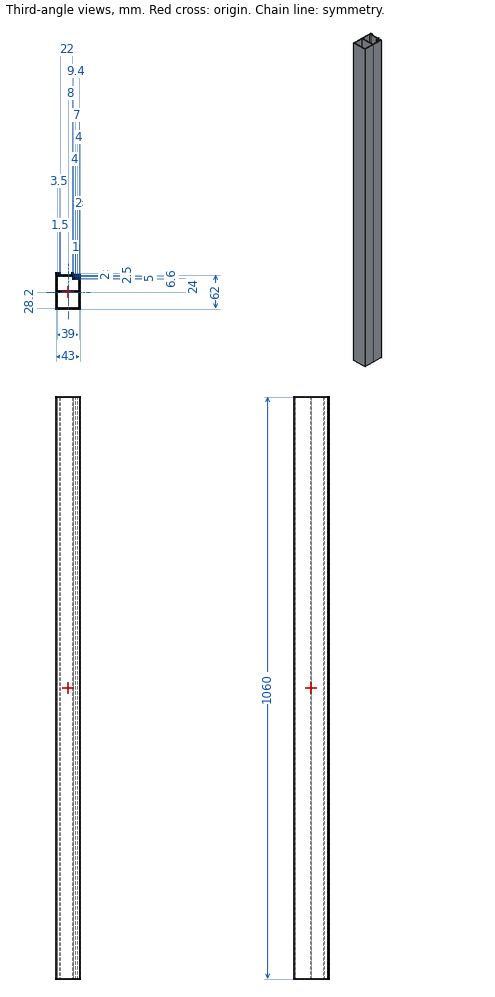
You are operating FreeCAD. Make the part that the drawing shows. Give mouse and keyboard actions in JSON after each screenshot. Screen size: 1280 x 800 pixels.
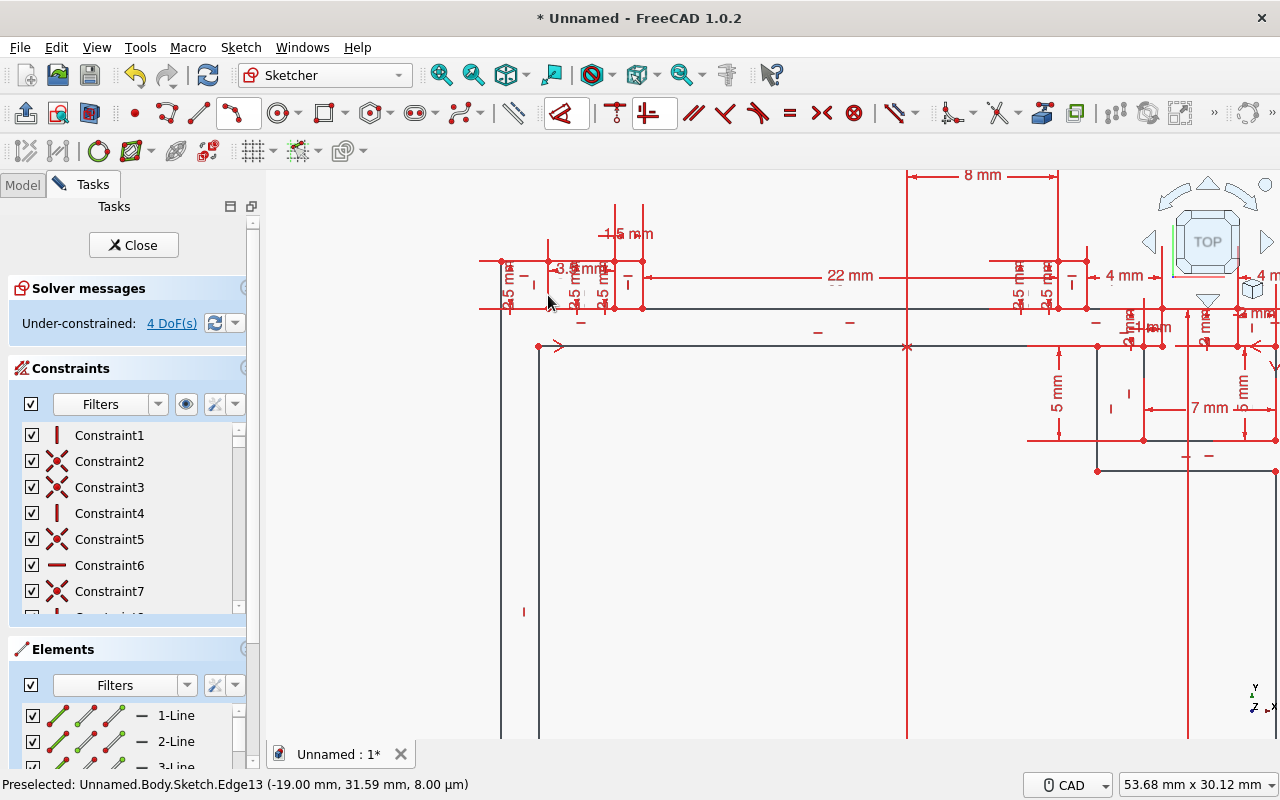
{"action": "left_click", "coordinate": [1097, 384]}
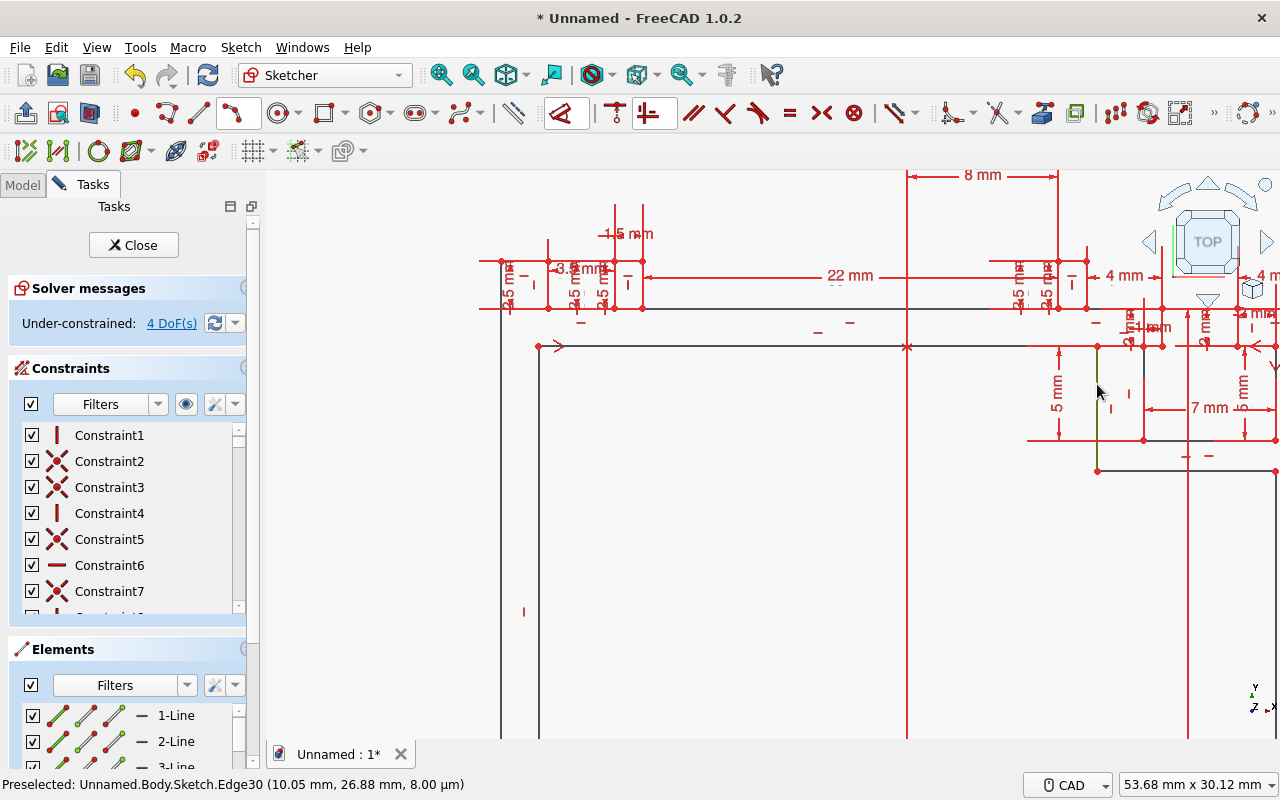
{"action": "left_click", "coordinate": [584, 114]}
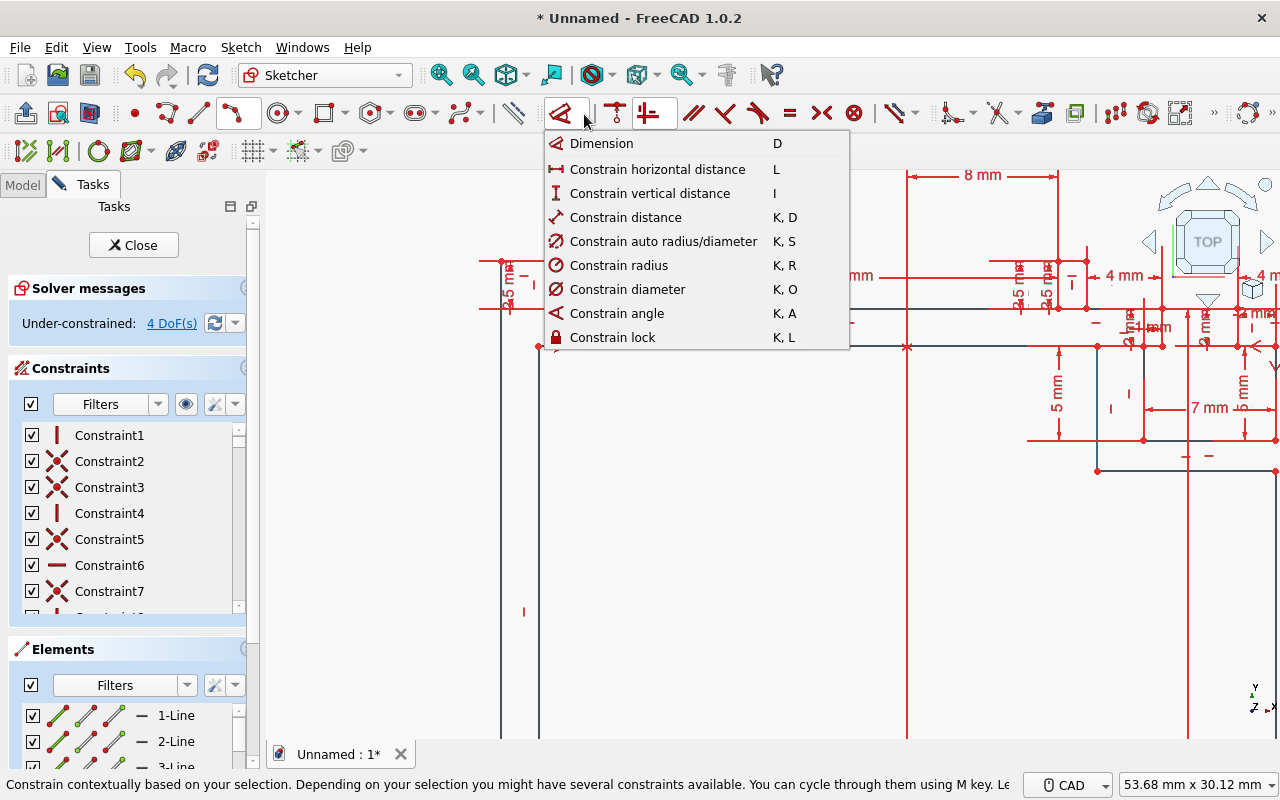
{"action": "left_click", "coordinate": [697, 193]}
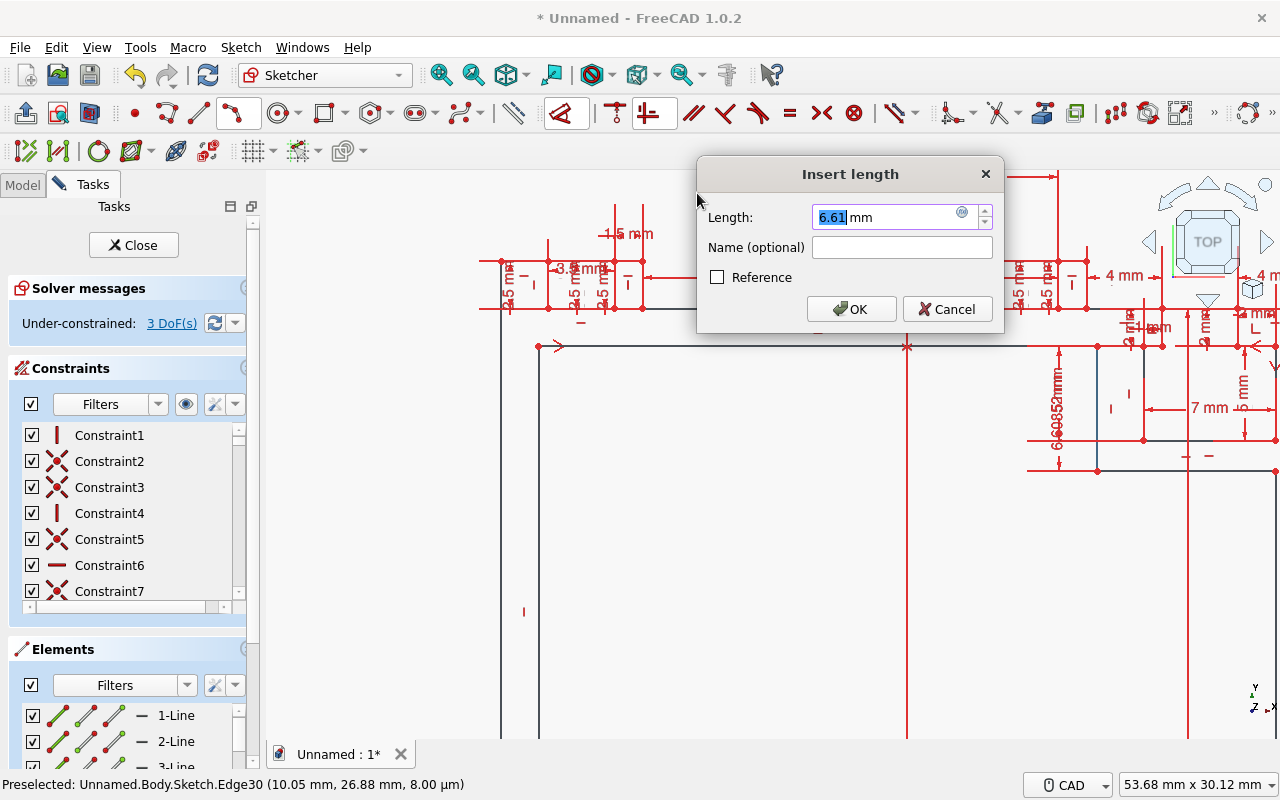
{"action": "type", "text": "6.6"}
{"action": "key", "text": "Return"}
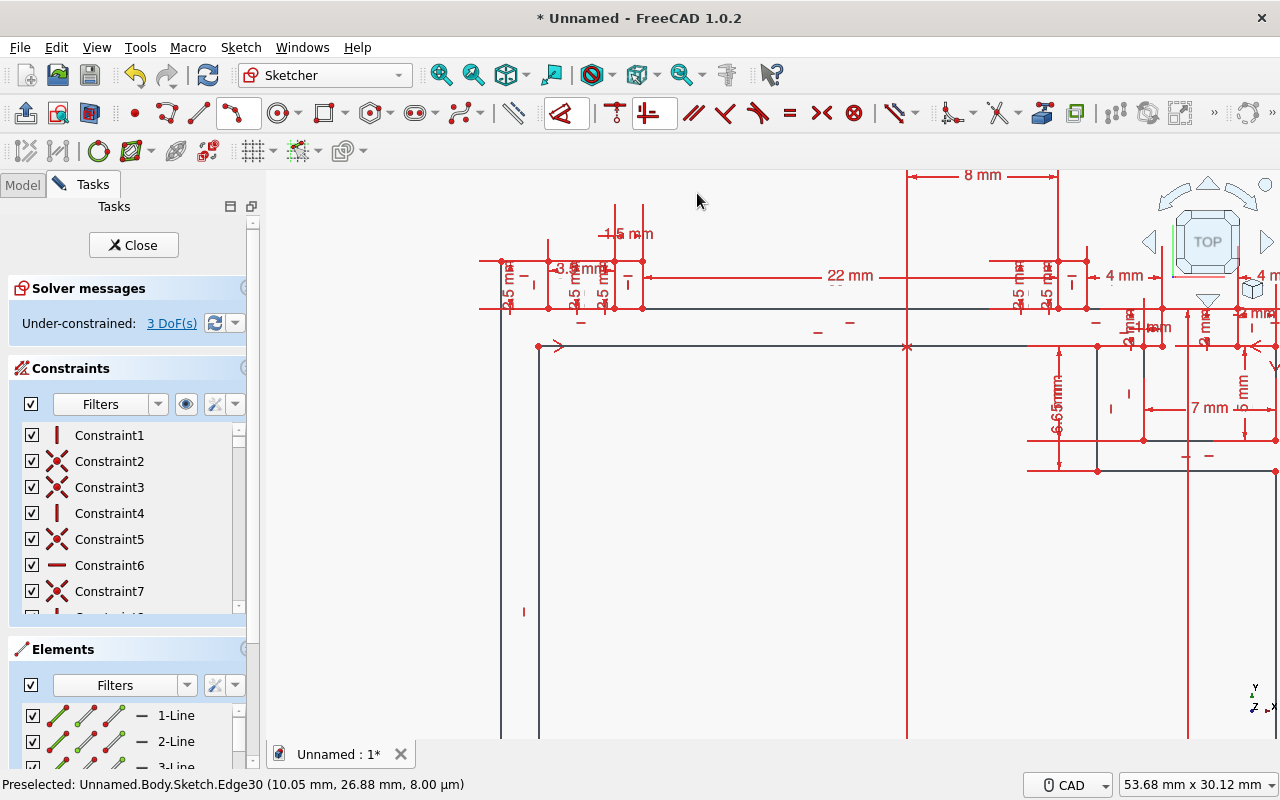
{"action": "scroll", "coordinate": [617, 276], "scroll_direction": "down", "scroll_amount": 6}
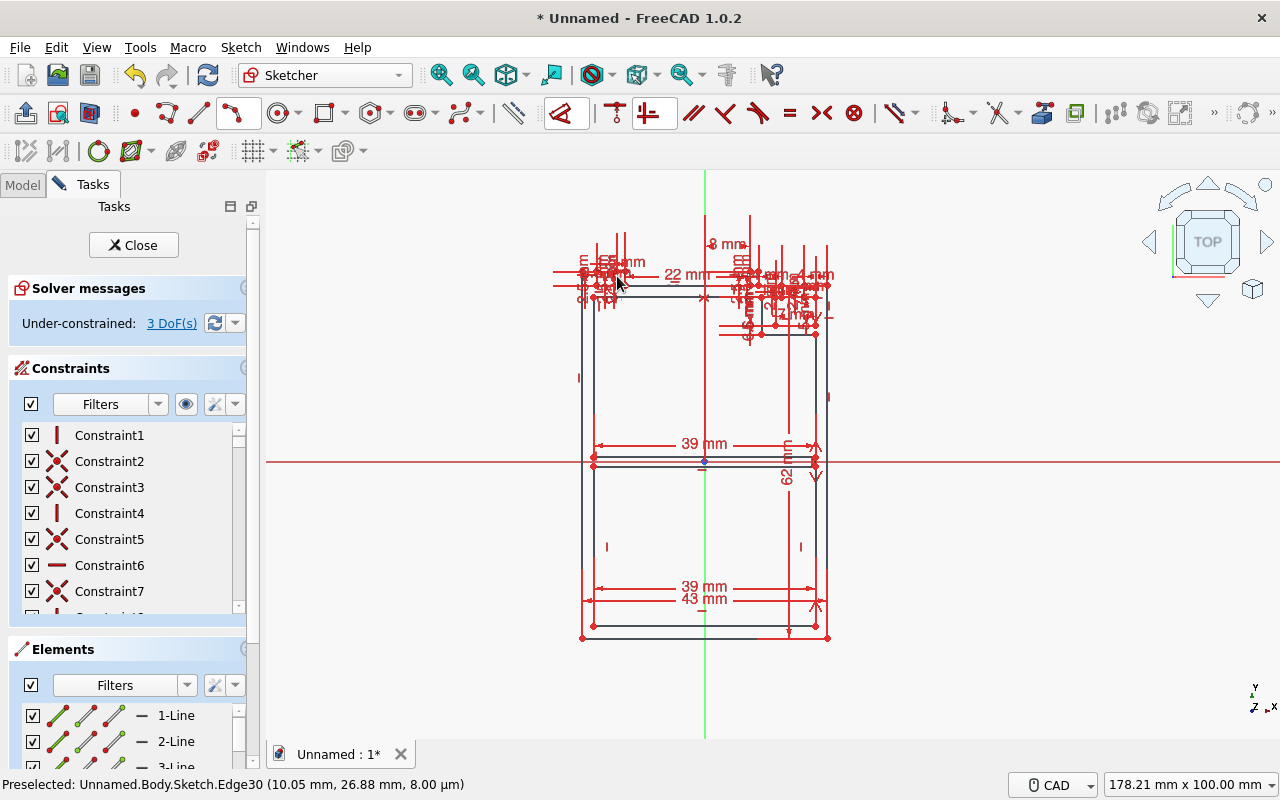
{"action": "scroll", "coordinate": [778, 335], "scroll_direction": "up", "scroll_amount": 3}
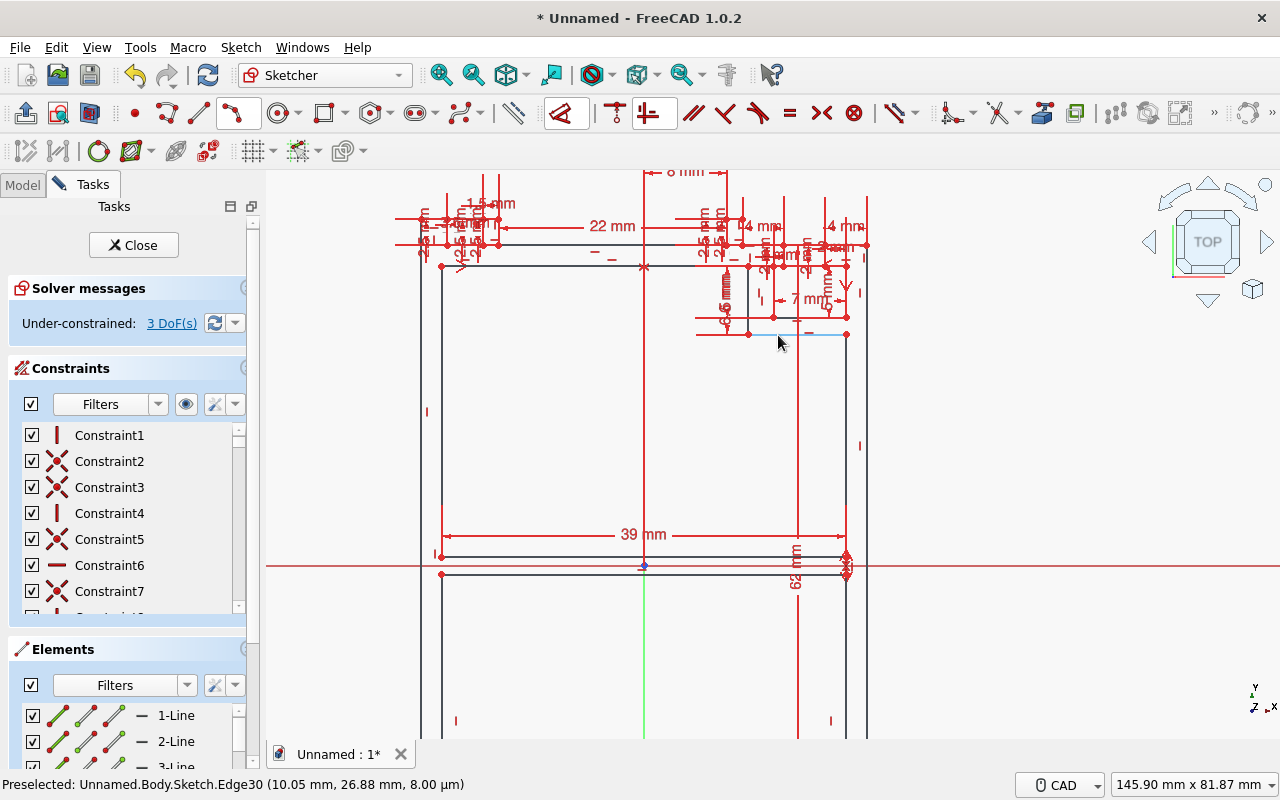
{"action": "left_click", "coordinate": [778, 335]}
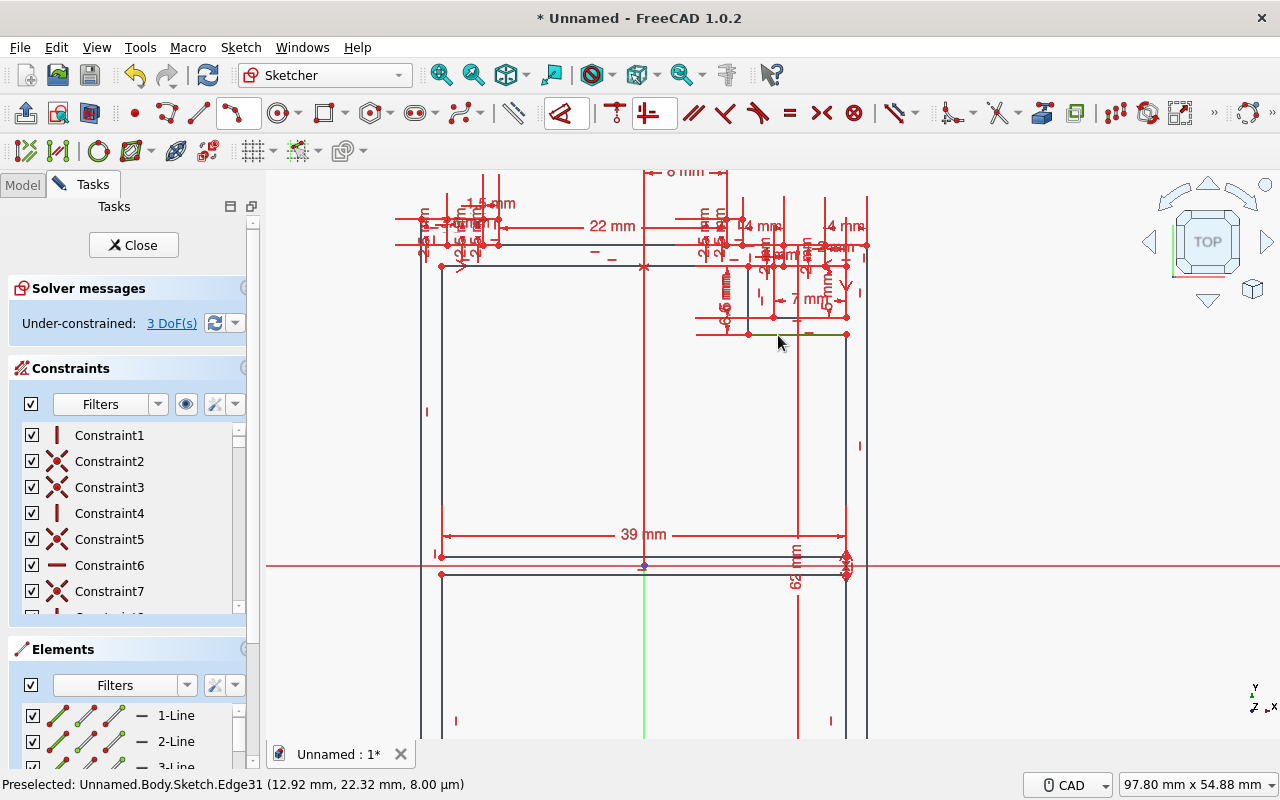
{"action": "key", "text": "l"}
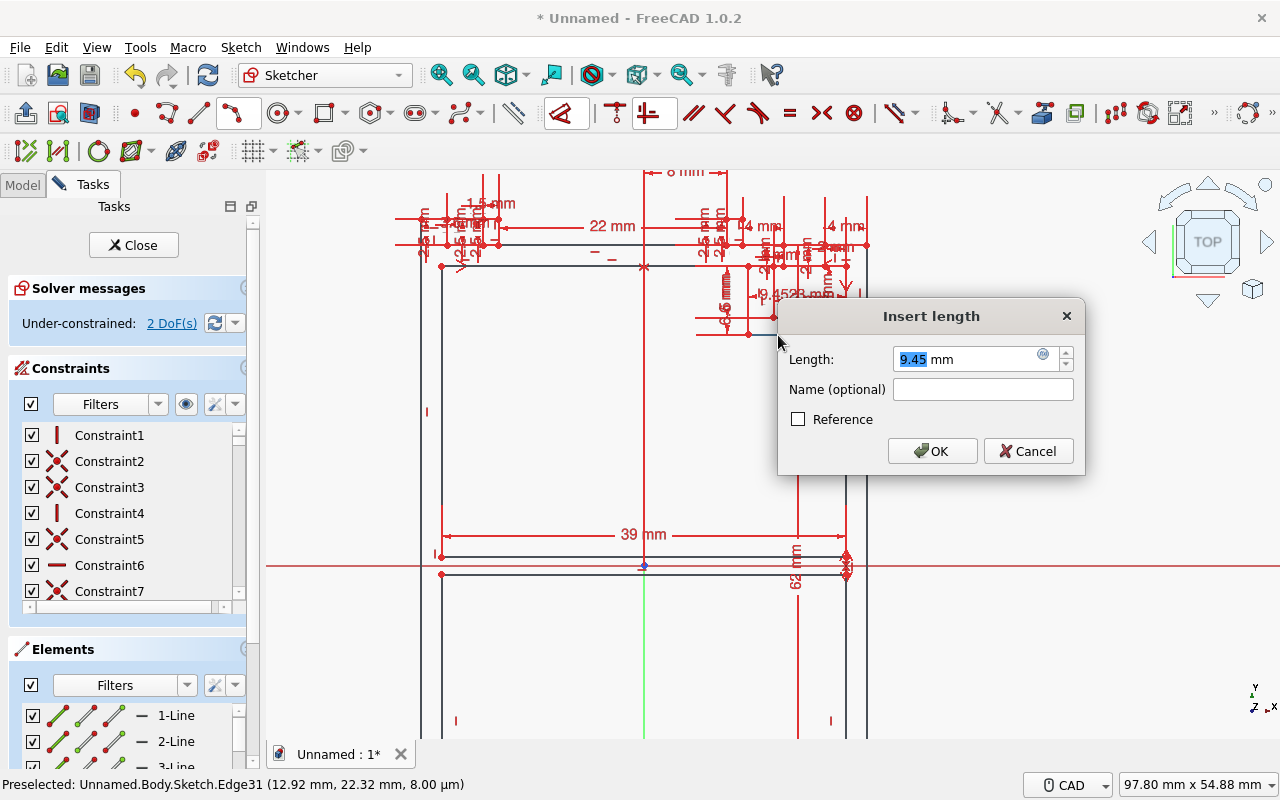
{"action": "type", "text": "9.4"}
{"action": "key", "text": "Return"}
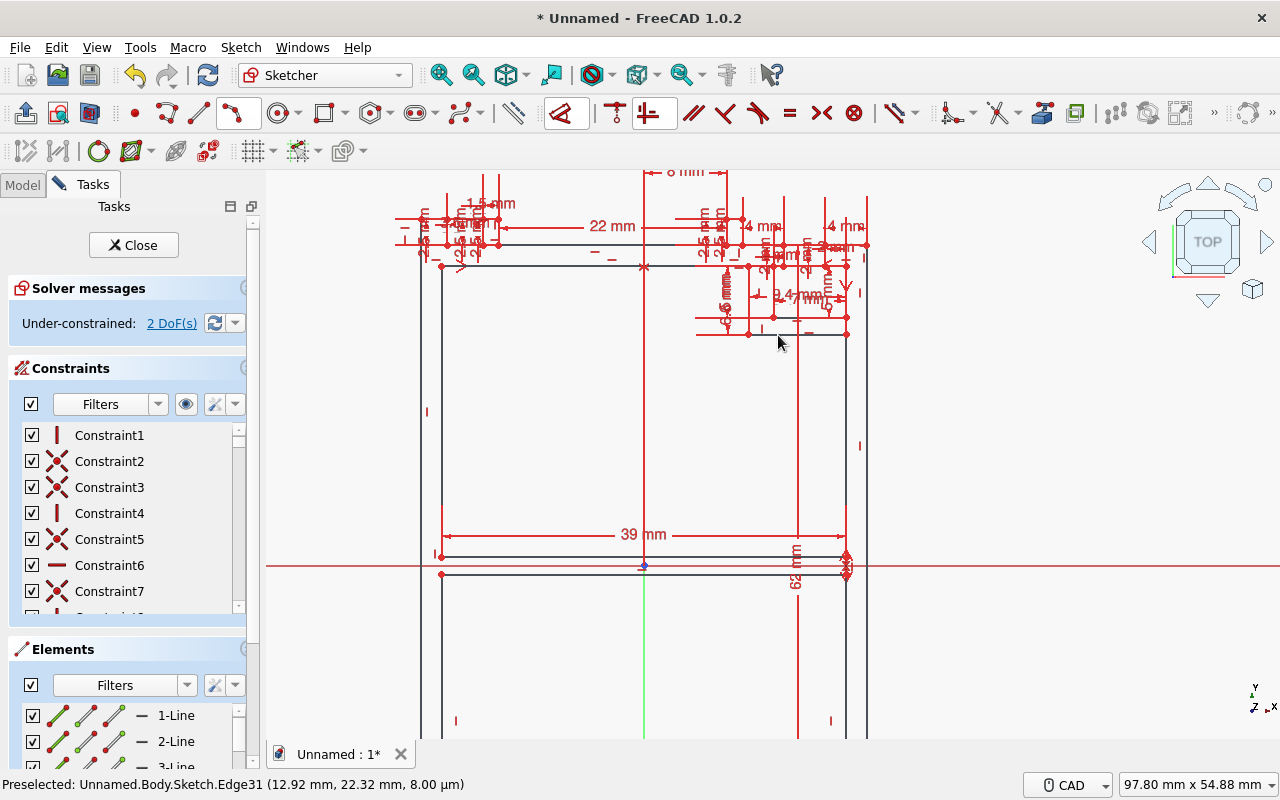
{"action": "left_click", "coordinate": [774, 318]}